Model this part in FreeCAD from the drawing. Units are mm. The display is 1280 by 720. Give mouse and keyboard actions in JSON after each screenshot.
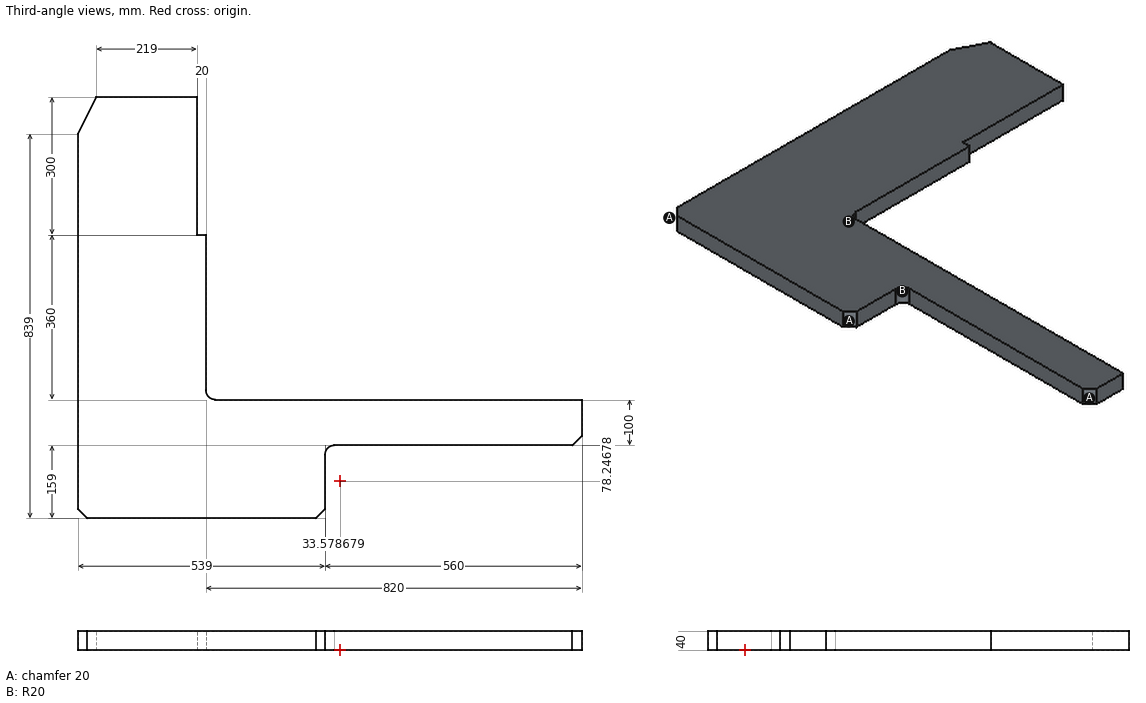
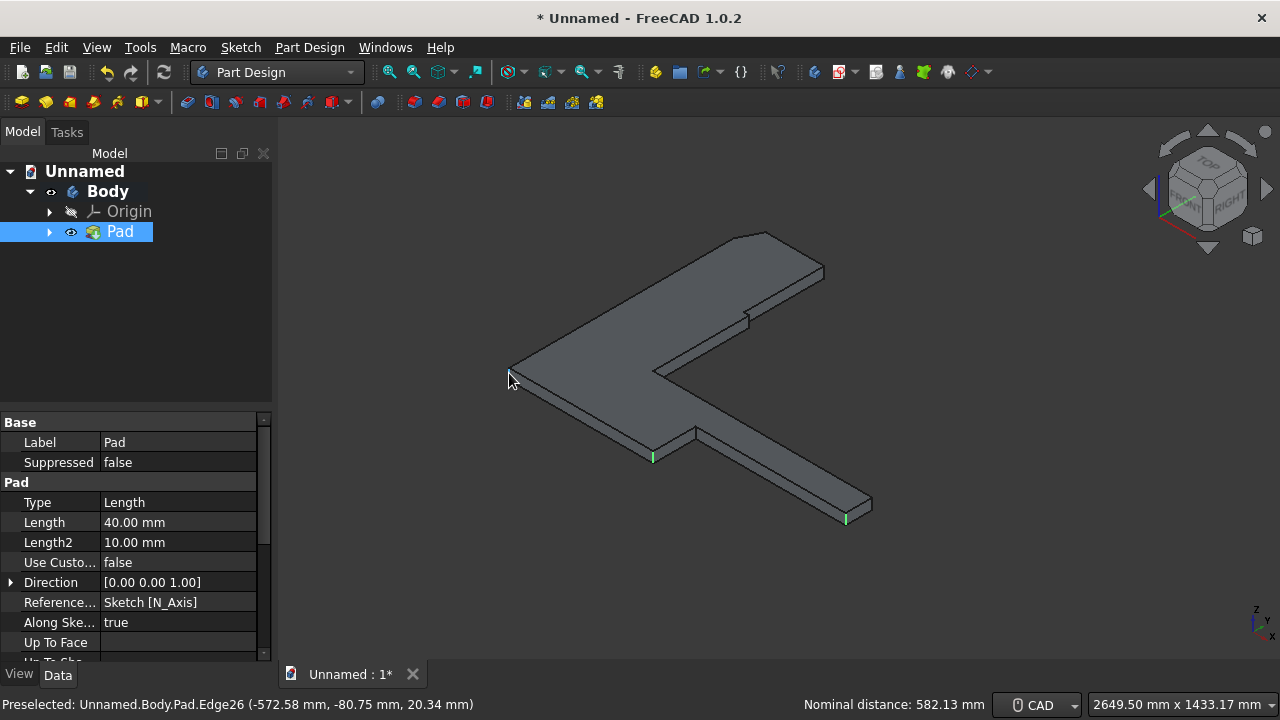
{"action": "key", "text": "2"}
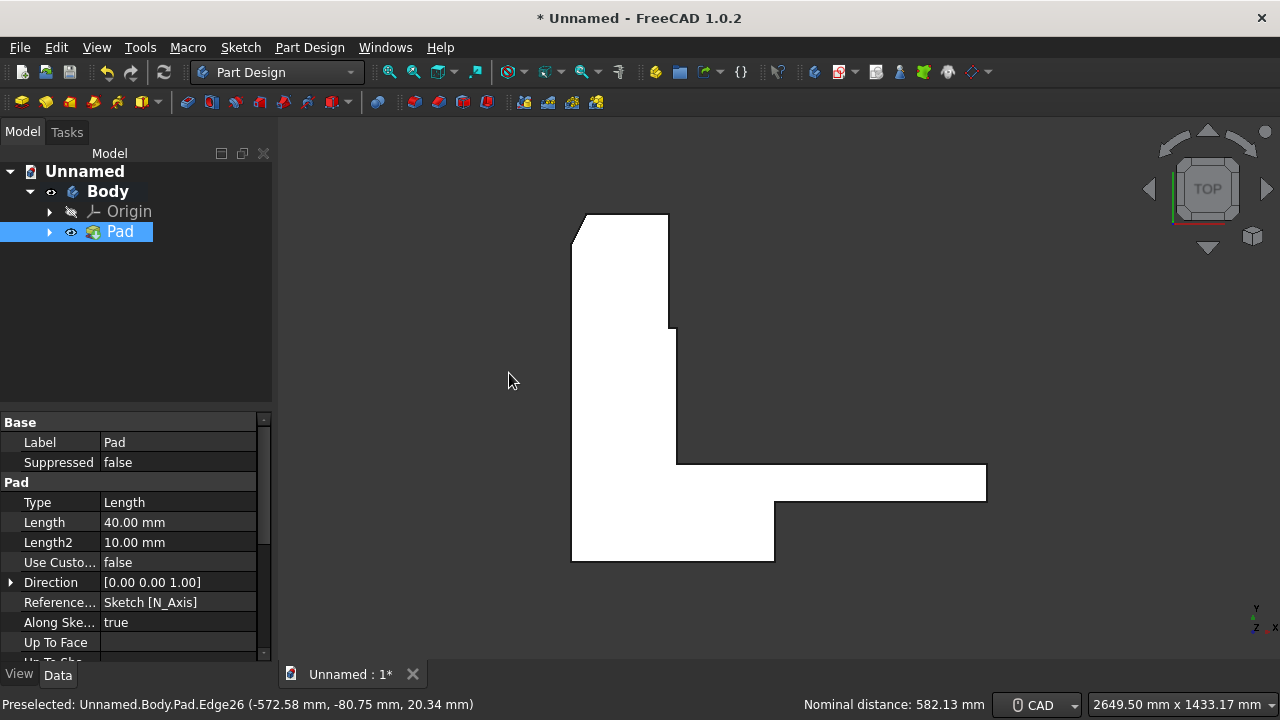
{"action": "scroll", "coordinate": [571, 561], "scroll_direction": "up", "scroll_amount": 5}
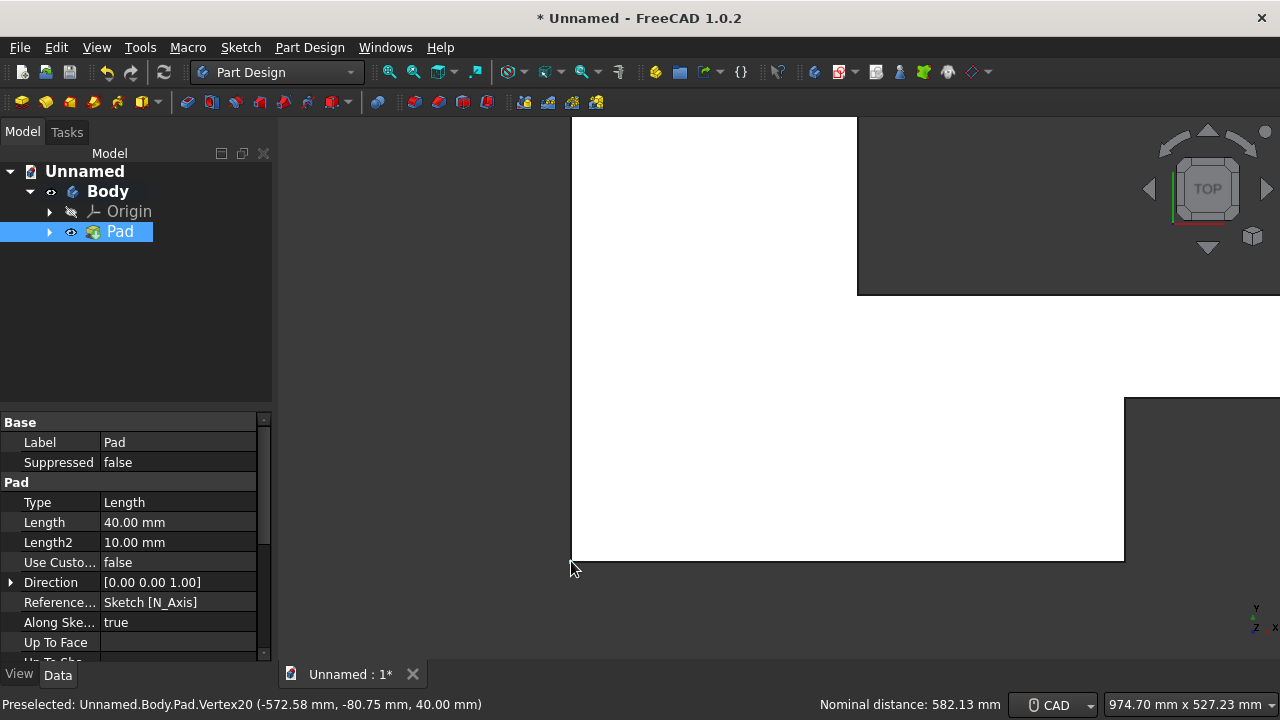
{"action": "key", "text": "v f"}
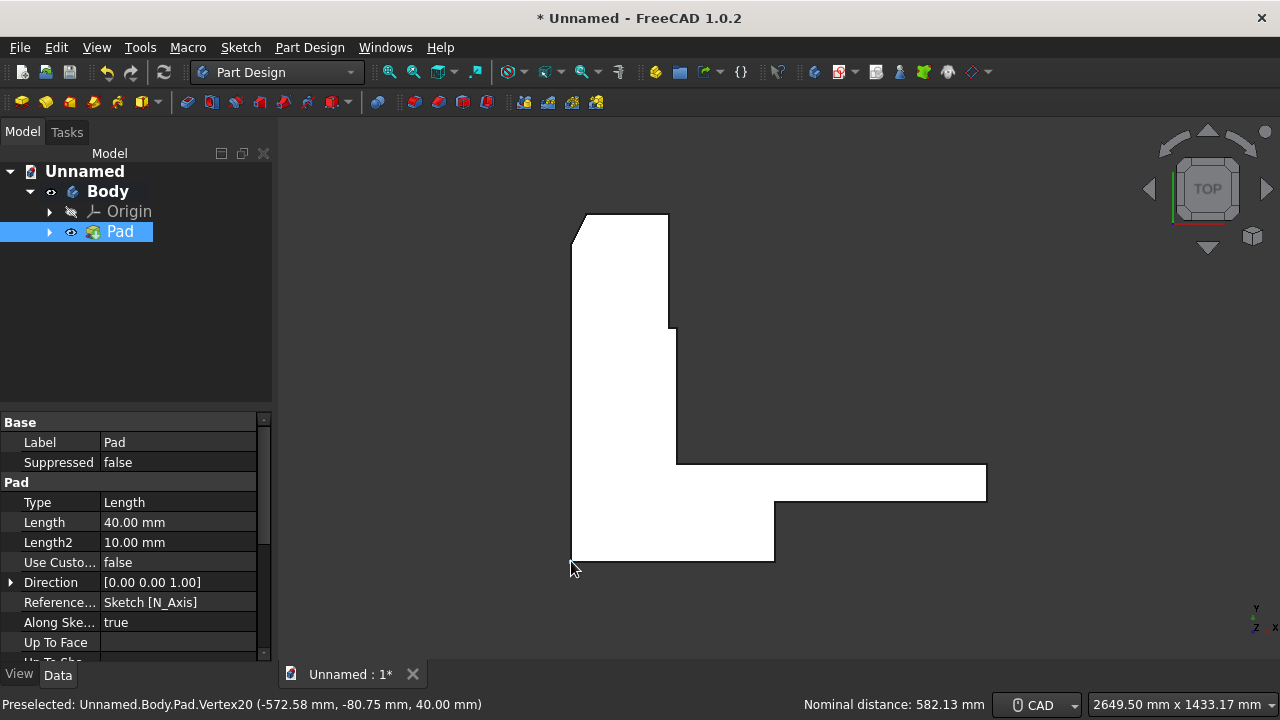
{"action": "key", "text": "1"}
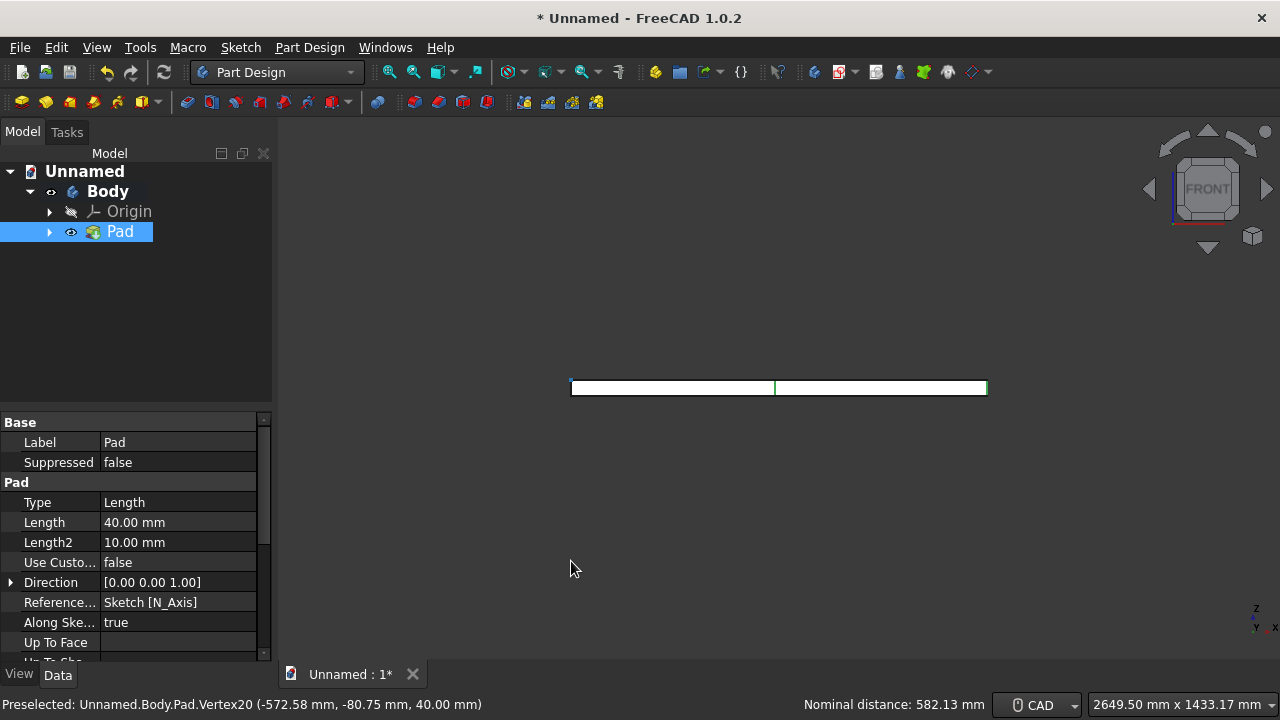
{"action": "key", "text": "v f"}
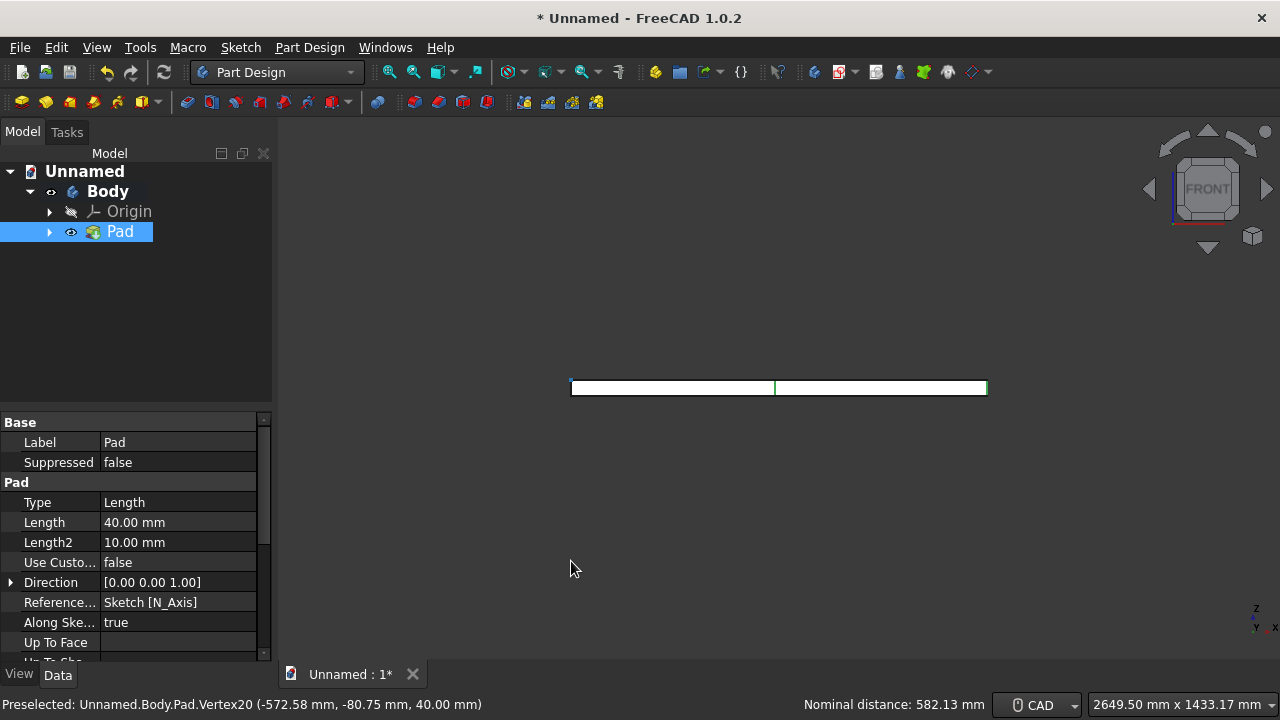
{"action": "left_click", "coordinate": [571, 387], "text": "ctrl"}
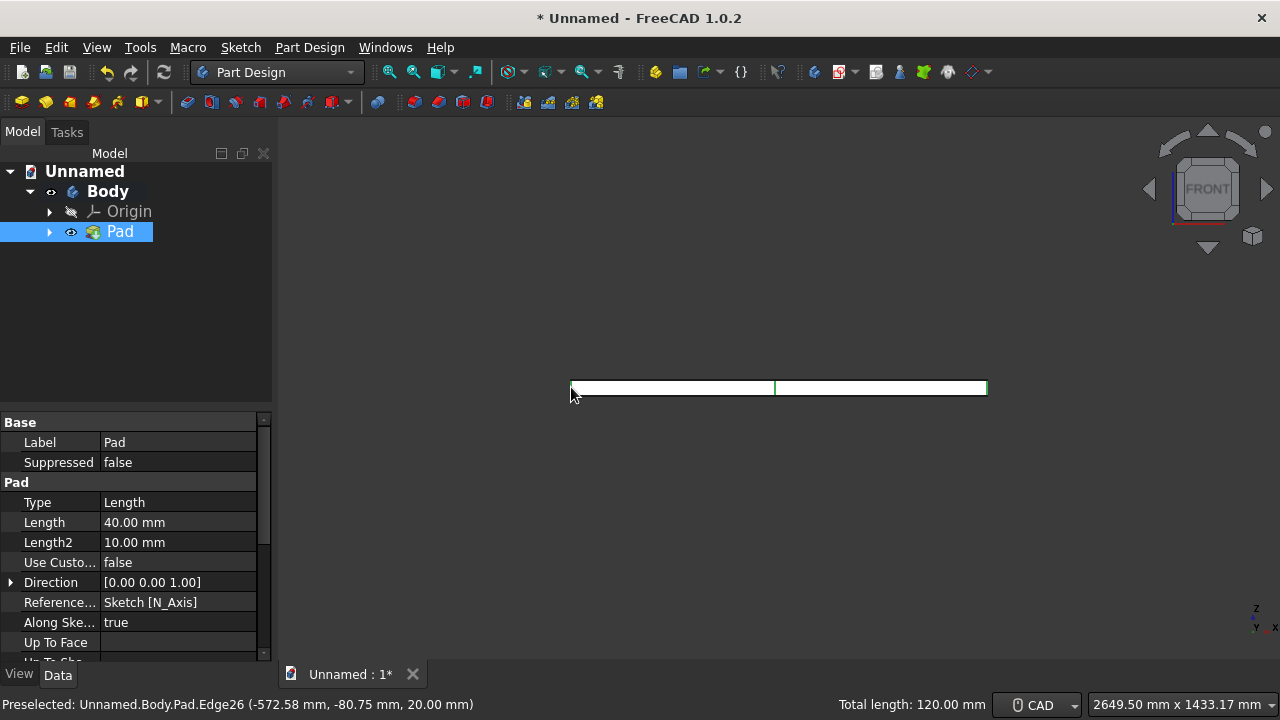
{"action": "left_click", "coordinate": [440, 102]}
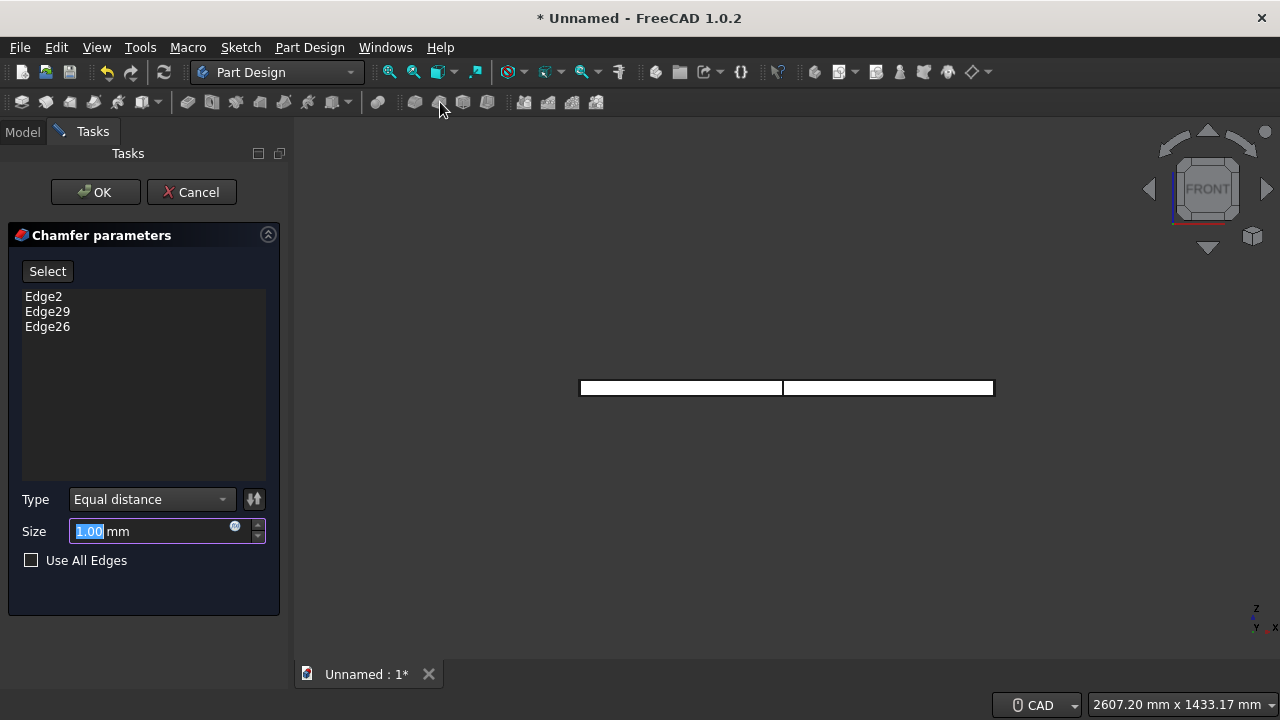
{"action": "type", "text": "20"}
{"action": "key", "text": "Tab"}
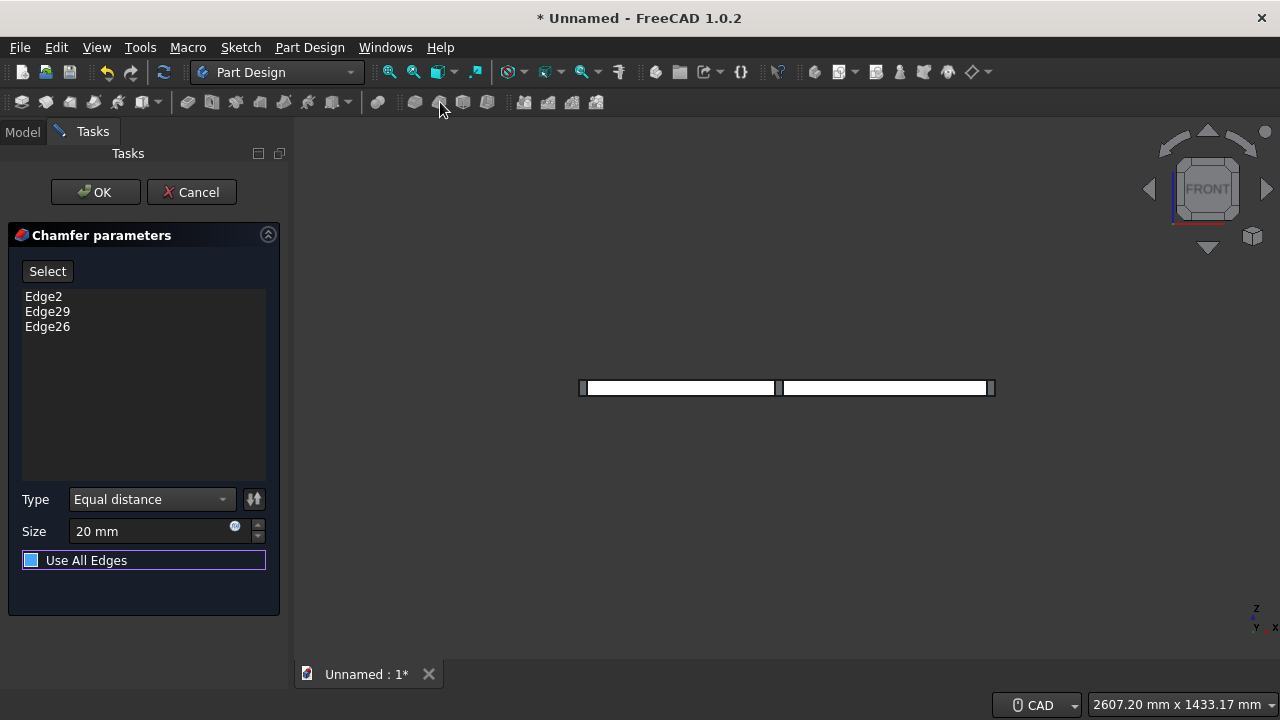
{"action": "left_click", "coordinate": [96, 192]}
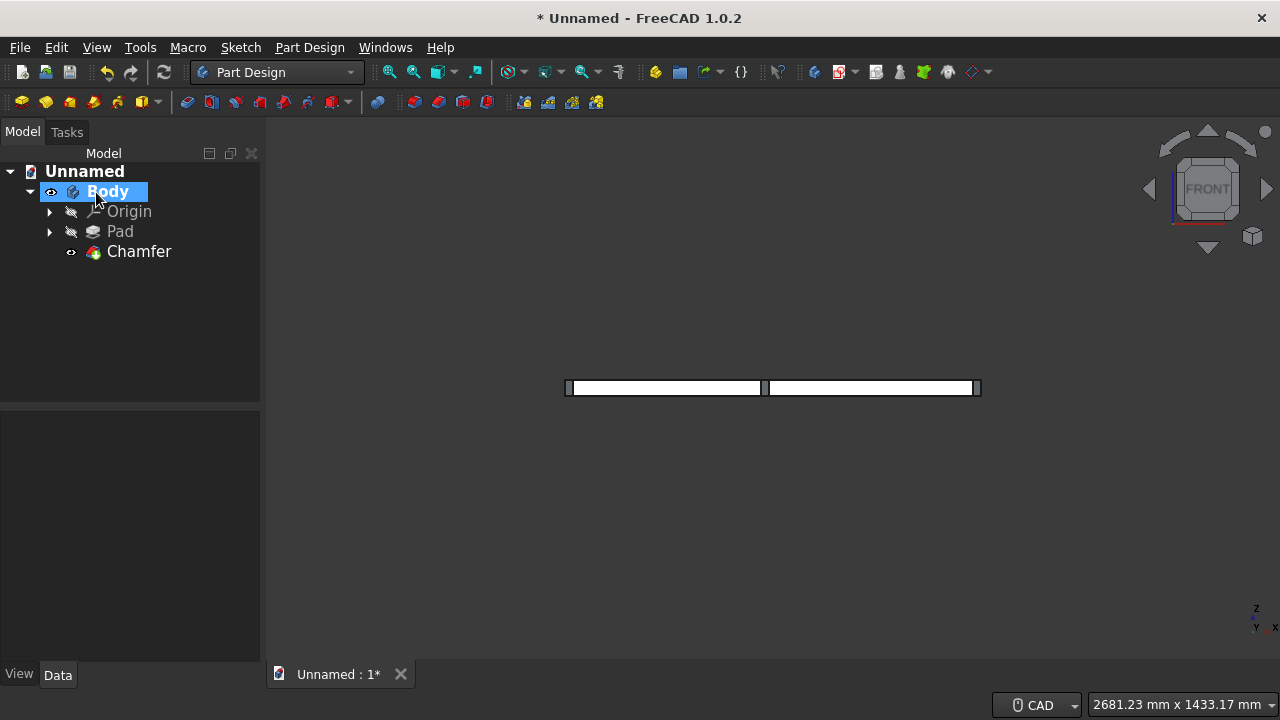
{"action": "key", "text": "v f"}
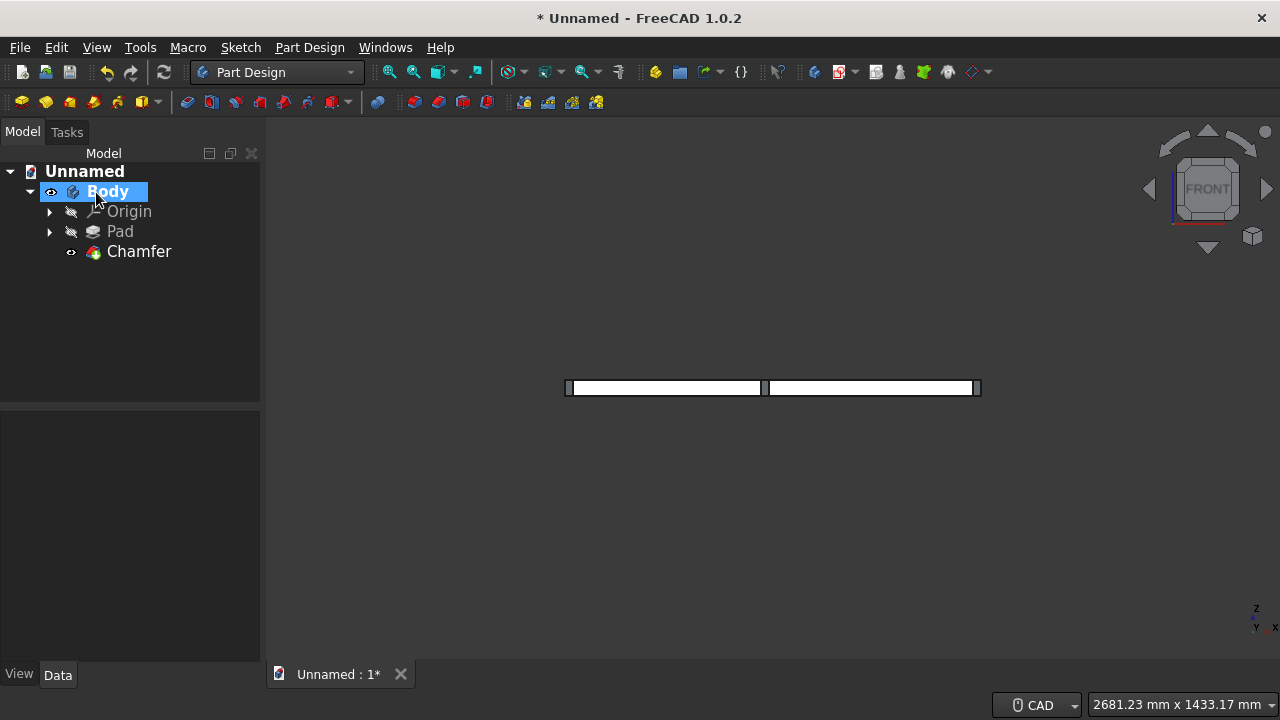
{"action": "scroll", "coordinate": [671, 387], "scroll_direction": "up", "scroll_amount": 5}